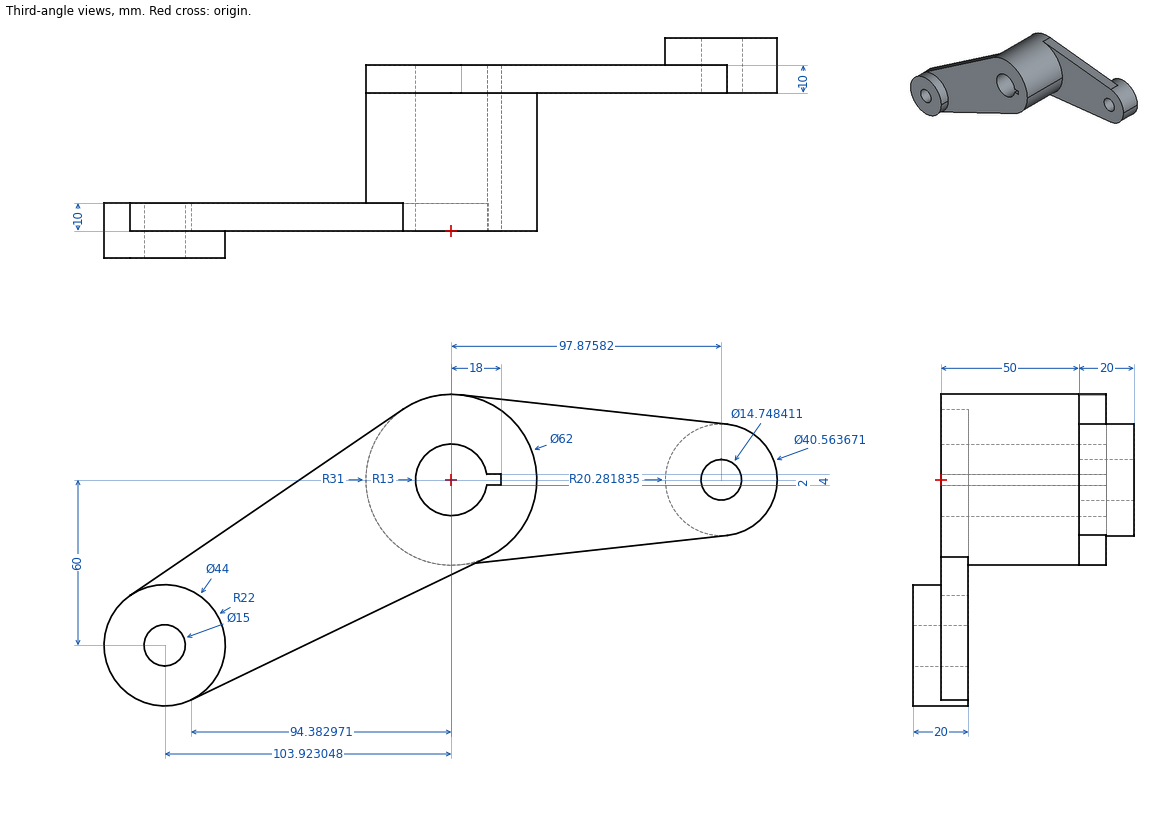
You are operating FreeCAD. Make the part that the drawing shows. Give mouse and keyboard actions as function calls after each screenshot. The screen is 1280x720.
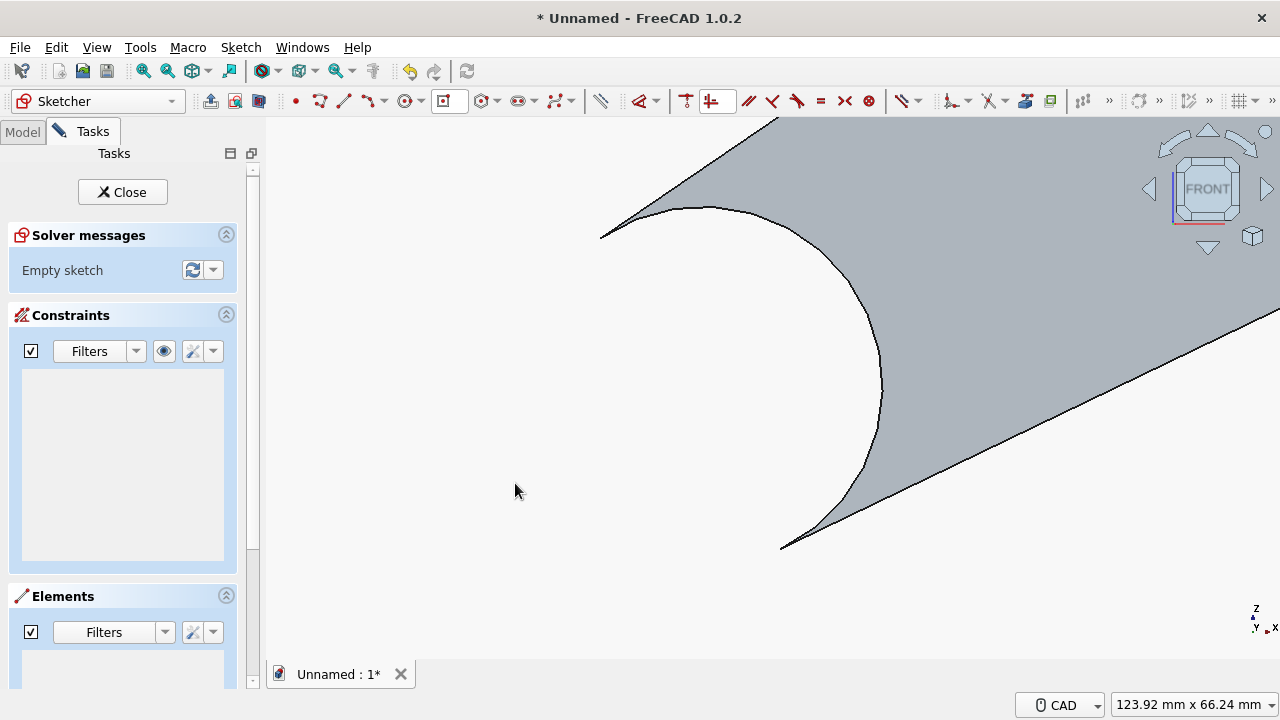
key(g)
key(c)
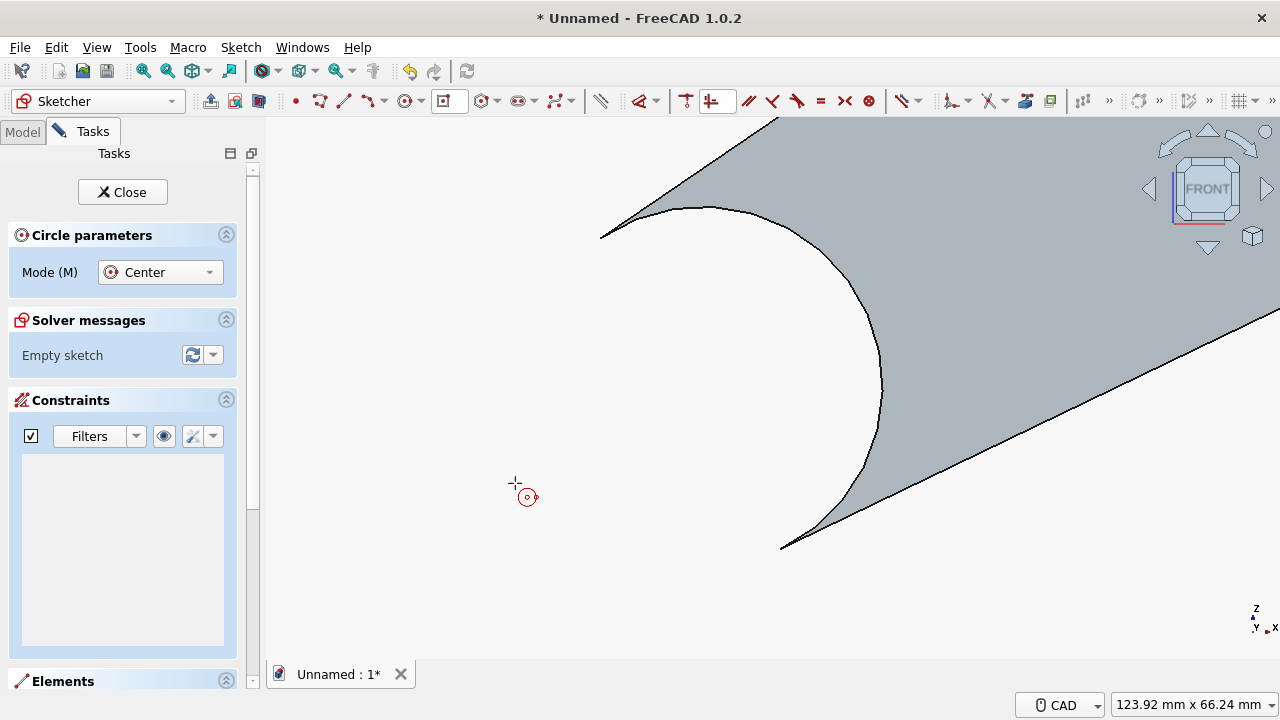
click(703, 387)
move(830, 259)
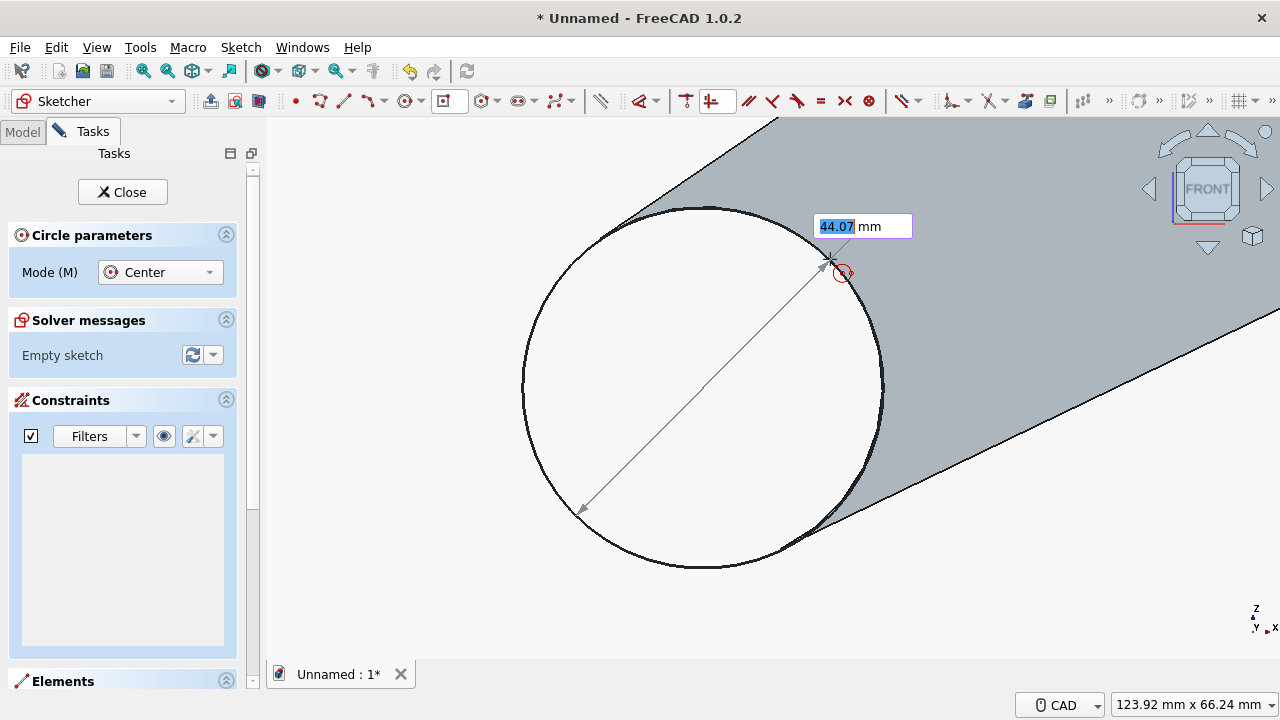
text(44)
key(Return)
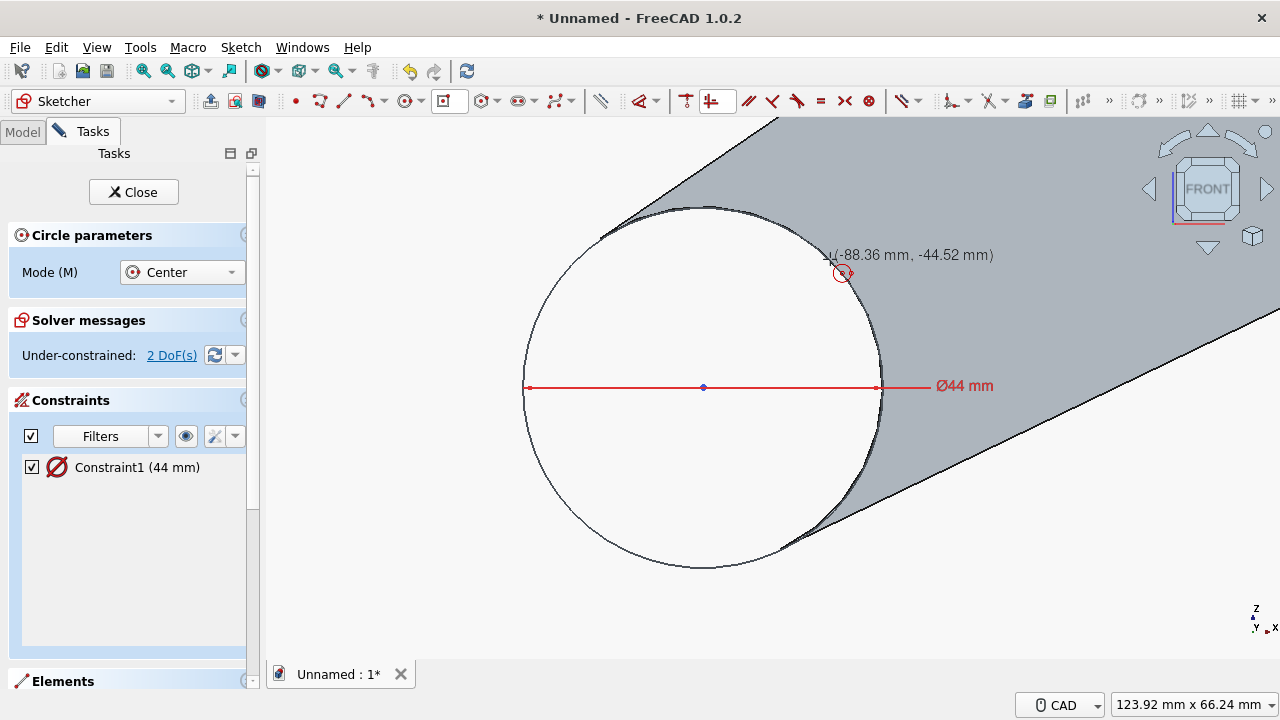
click(703, 388)
move(746, 343)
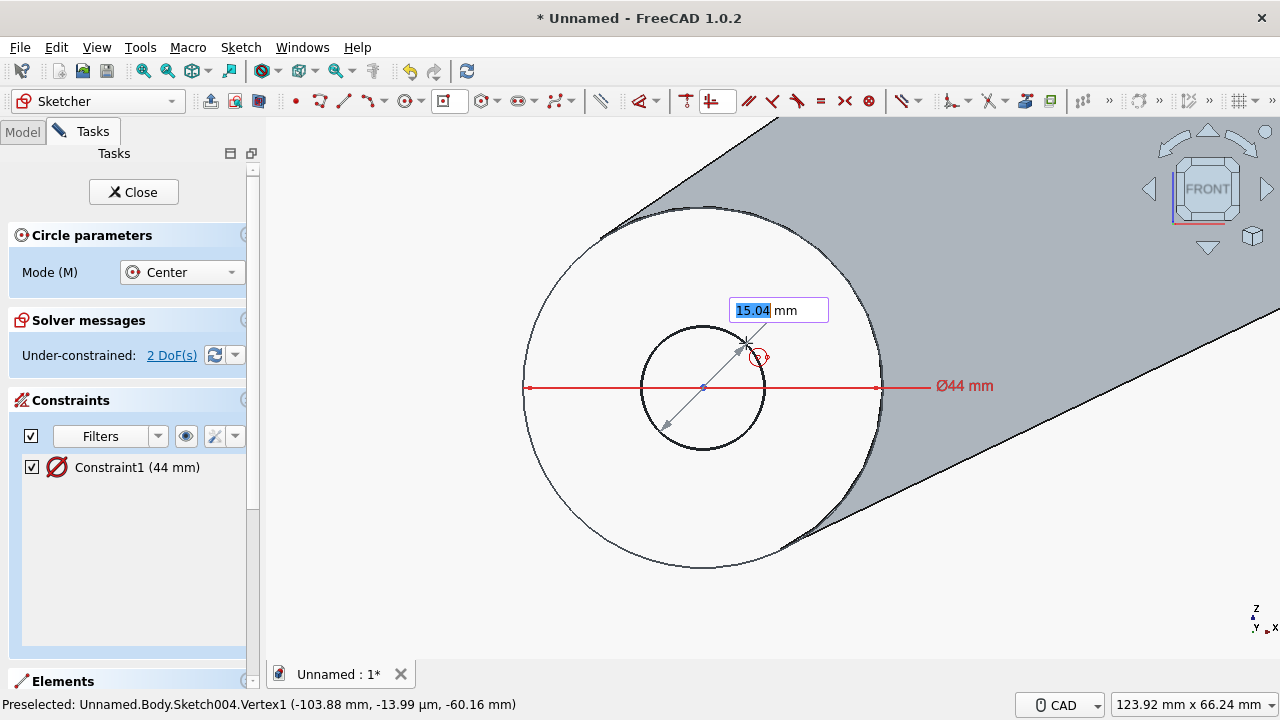
text(15)
key(Return)
key(Escape)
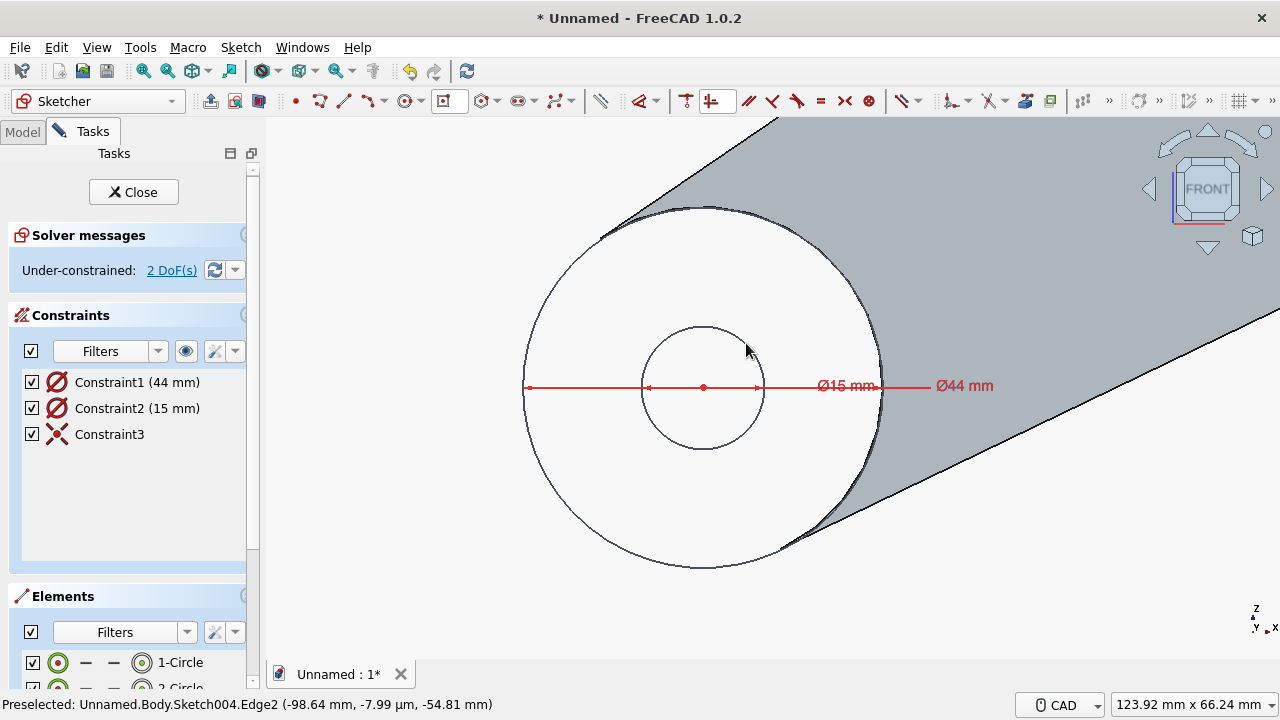
click(640, 102)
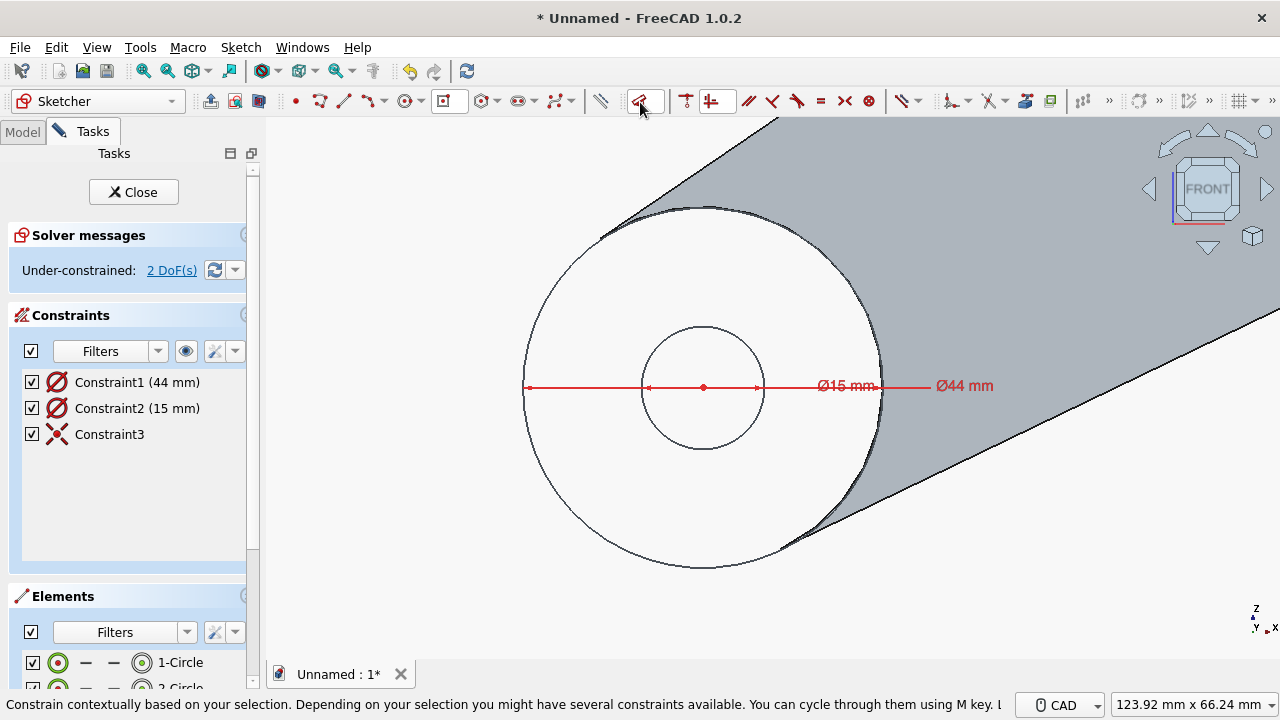
click(703, 388)
click(669, 267)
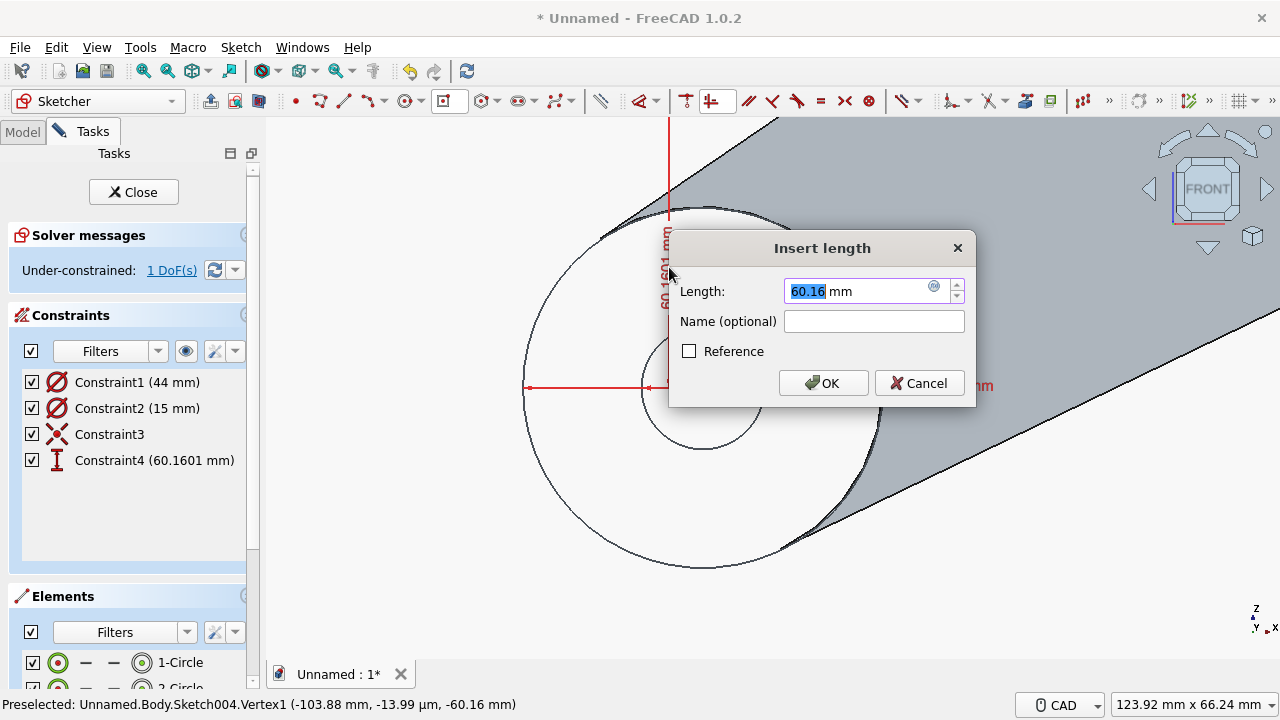
text(60)
key(Return)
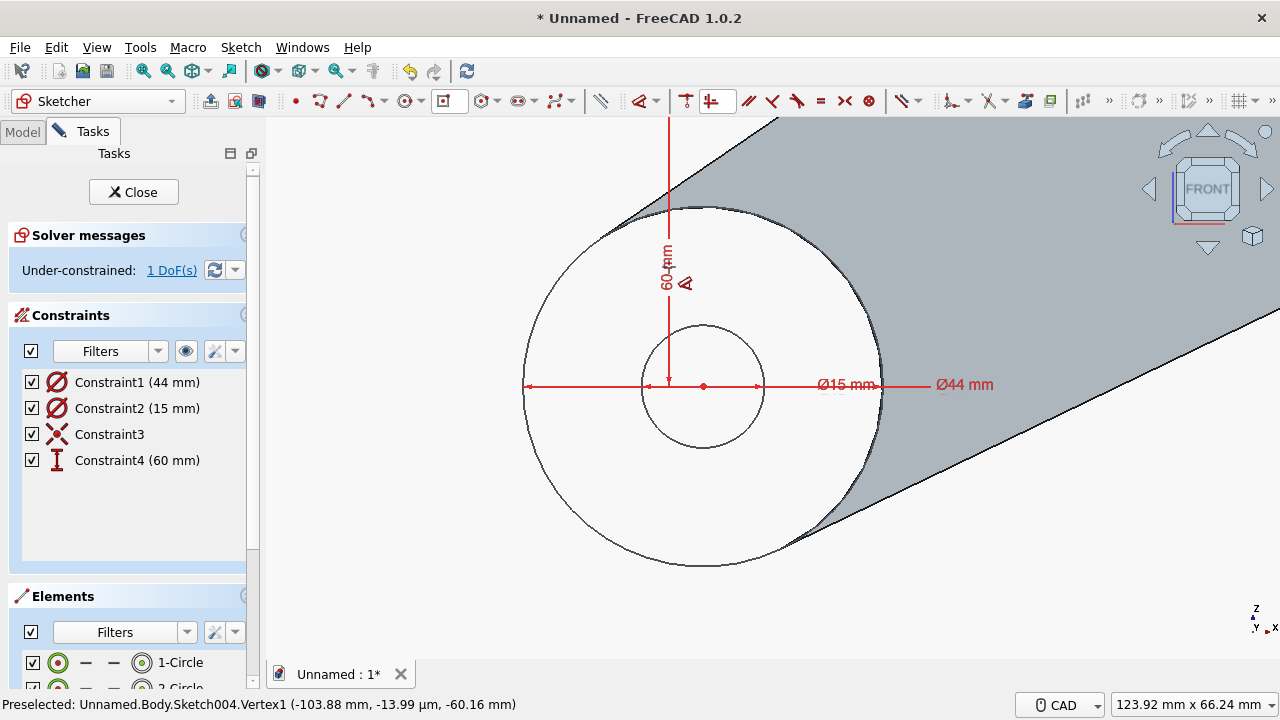
click(703, 387)
click(909, 421)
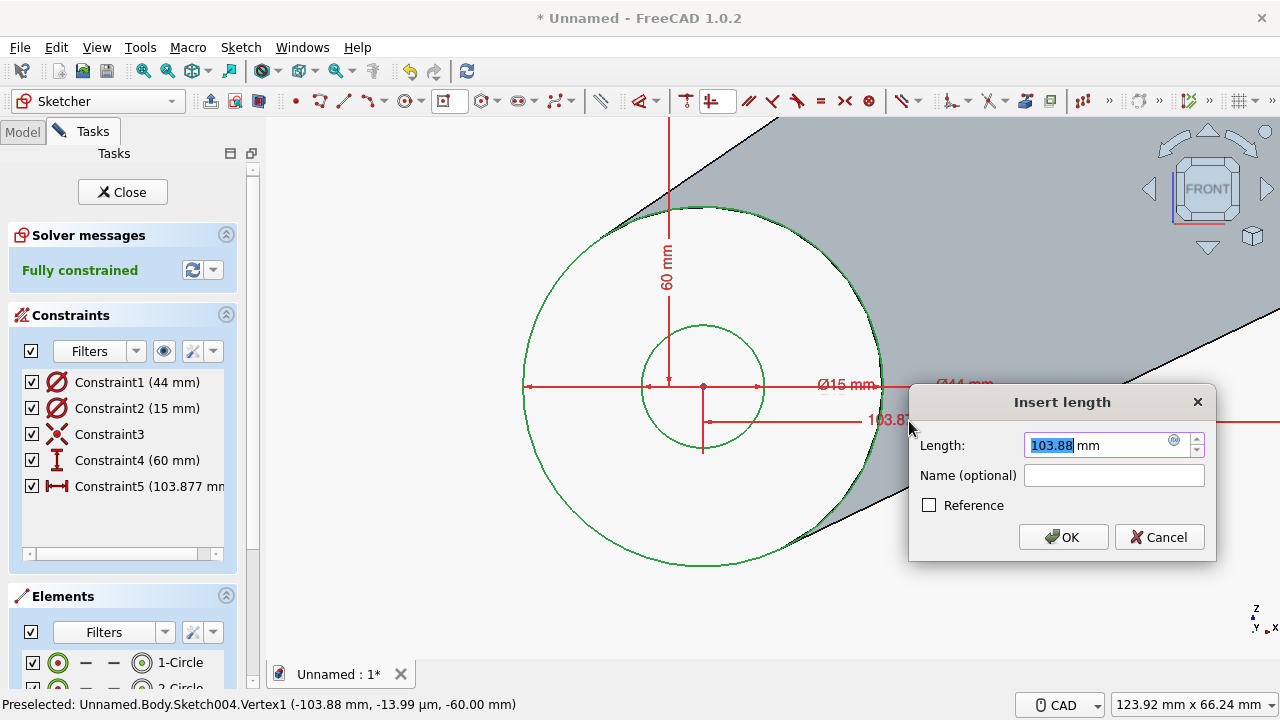
text(103.923048)
key(Return)
key(Escape)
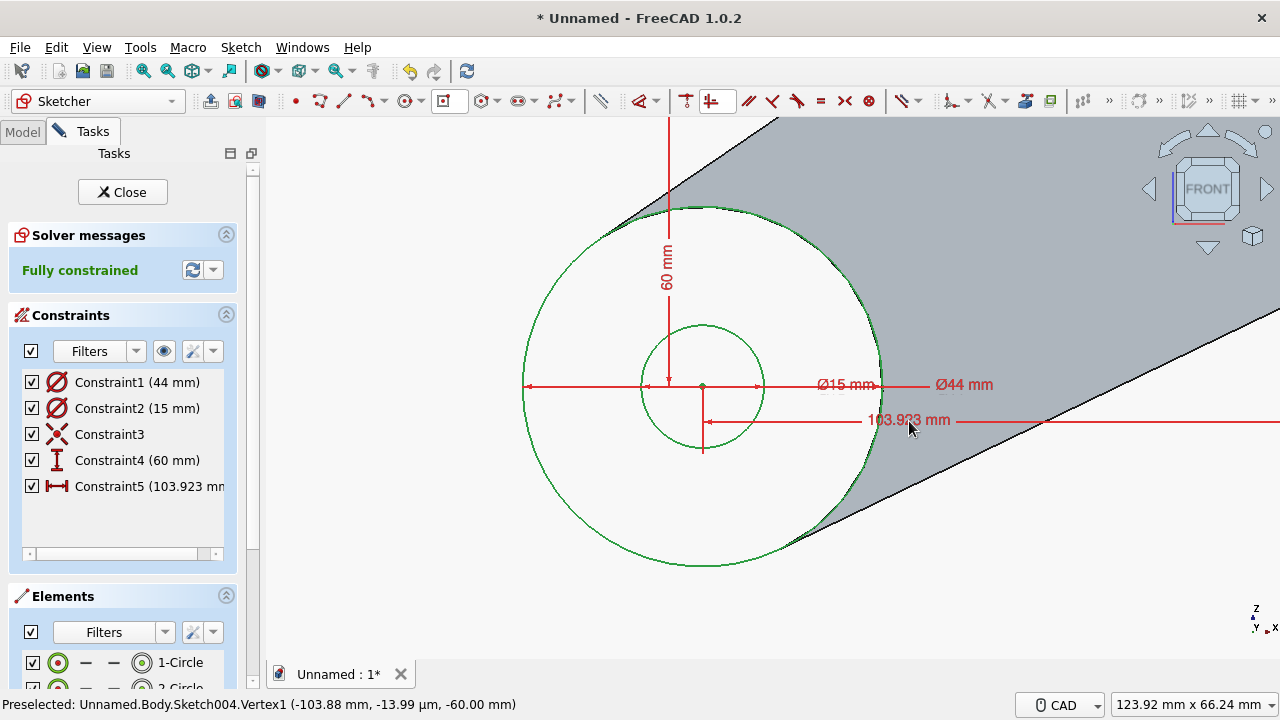
click(123, 192)